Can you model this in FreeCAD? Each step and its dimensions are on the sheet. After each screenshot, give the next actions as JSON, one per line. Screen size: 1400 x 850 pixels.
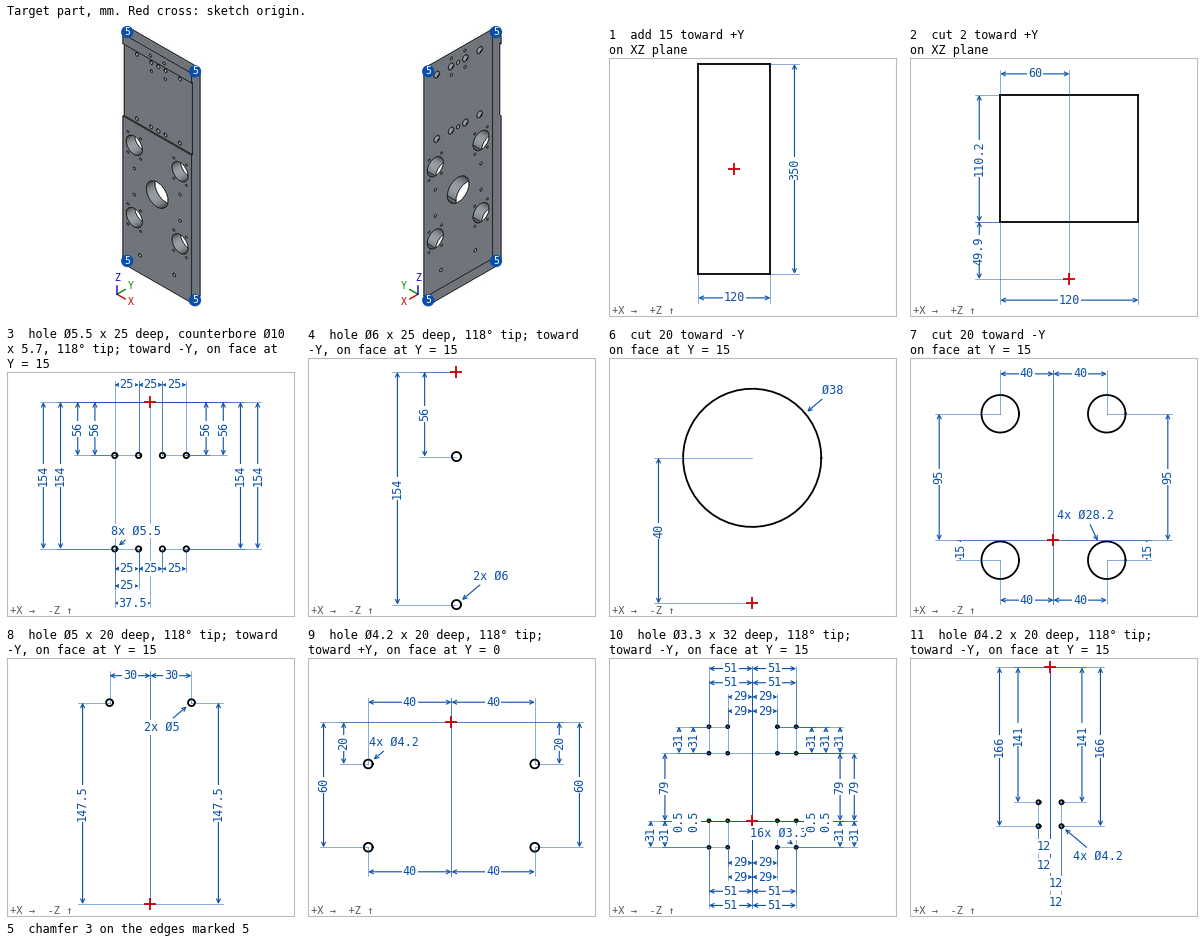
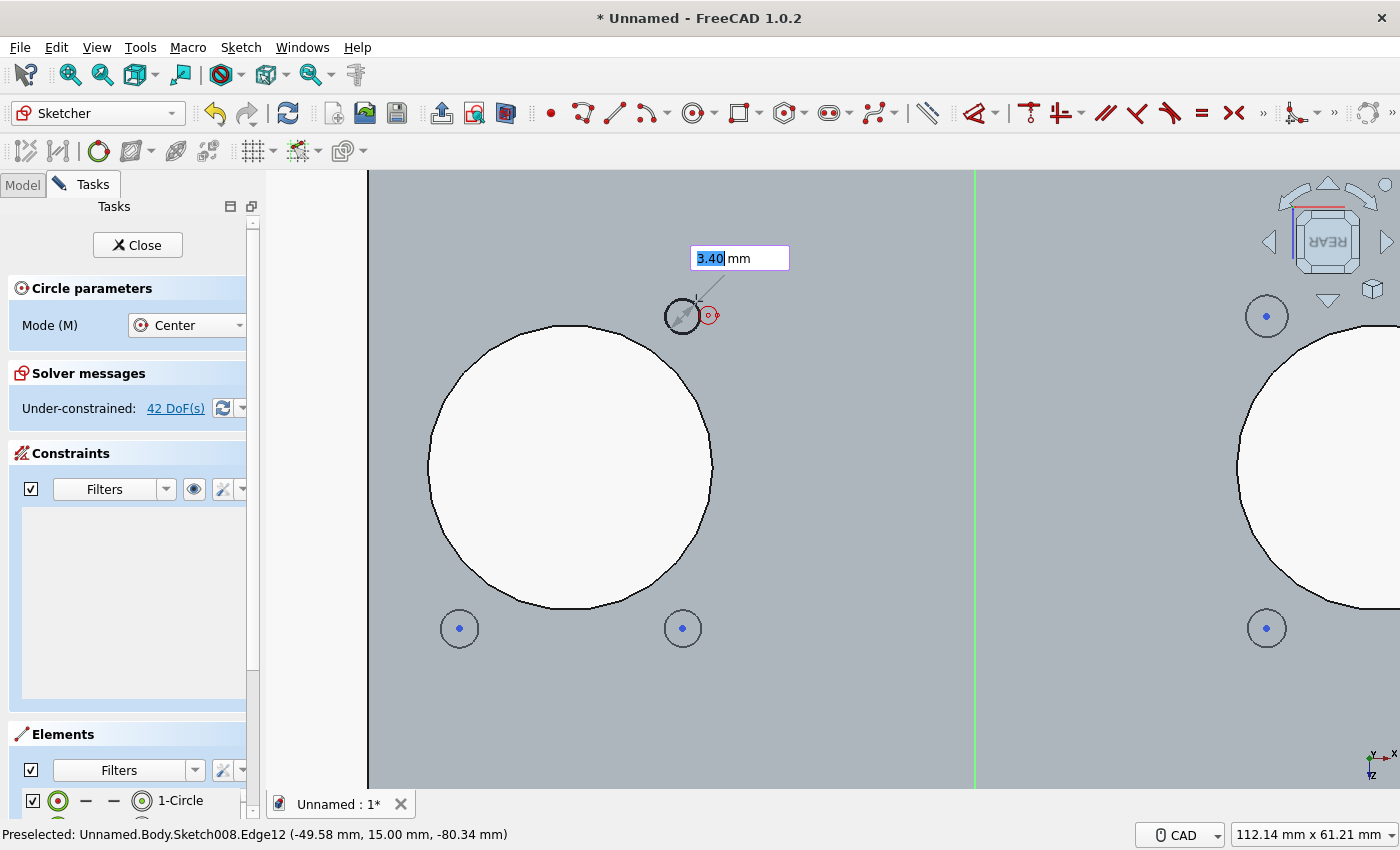
{"action": "left_click", "coordinate": [693, 299]}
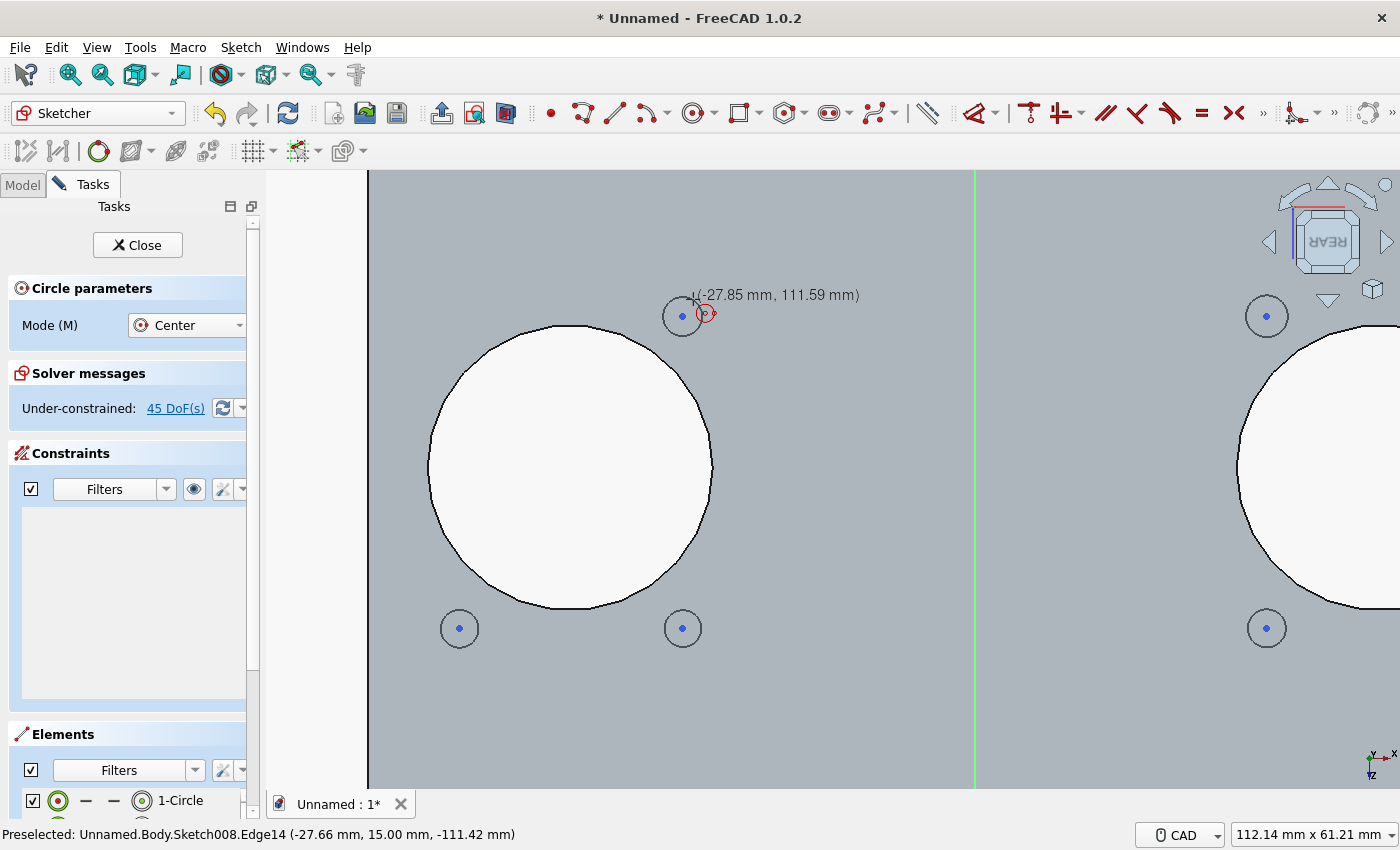
{"action": "scroll", "coordinate": [459, 311], "scroll_direction": "up", "scroll_amount": 2}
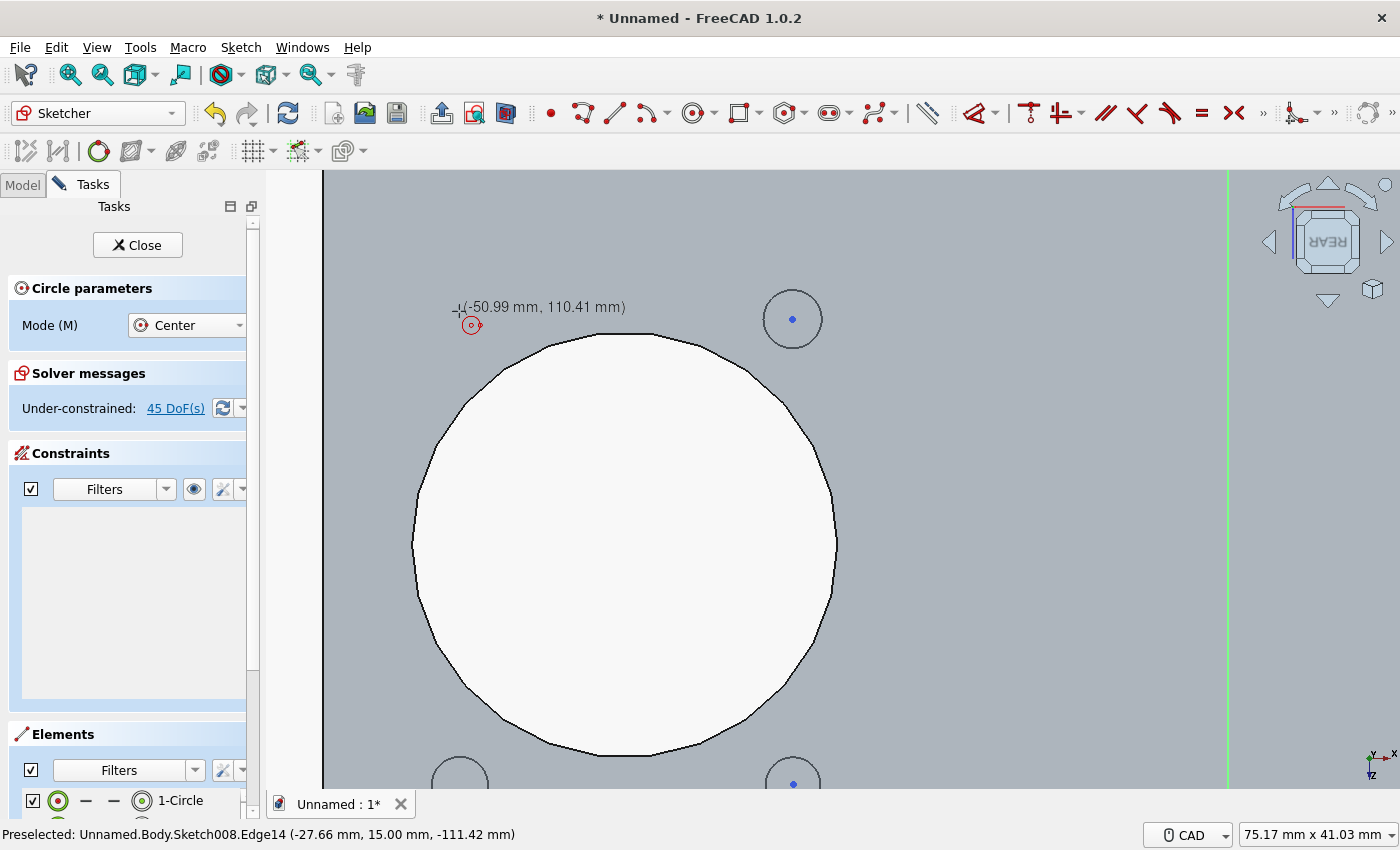
{"action": "scroll", "coordinate": [673, 302], "scroll_direction": "down", "scroll_amount": 9}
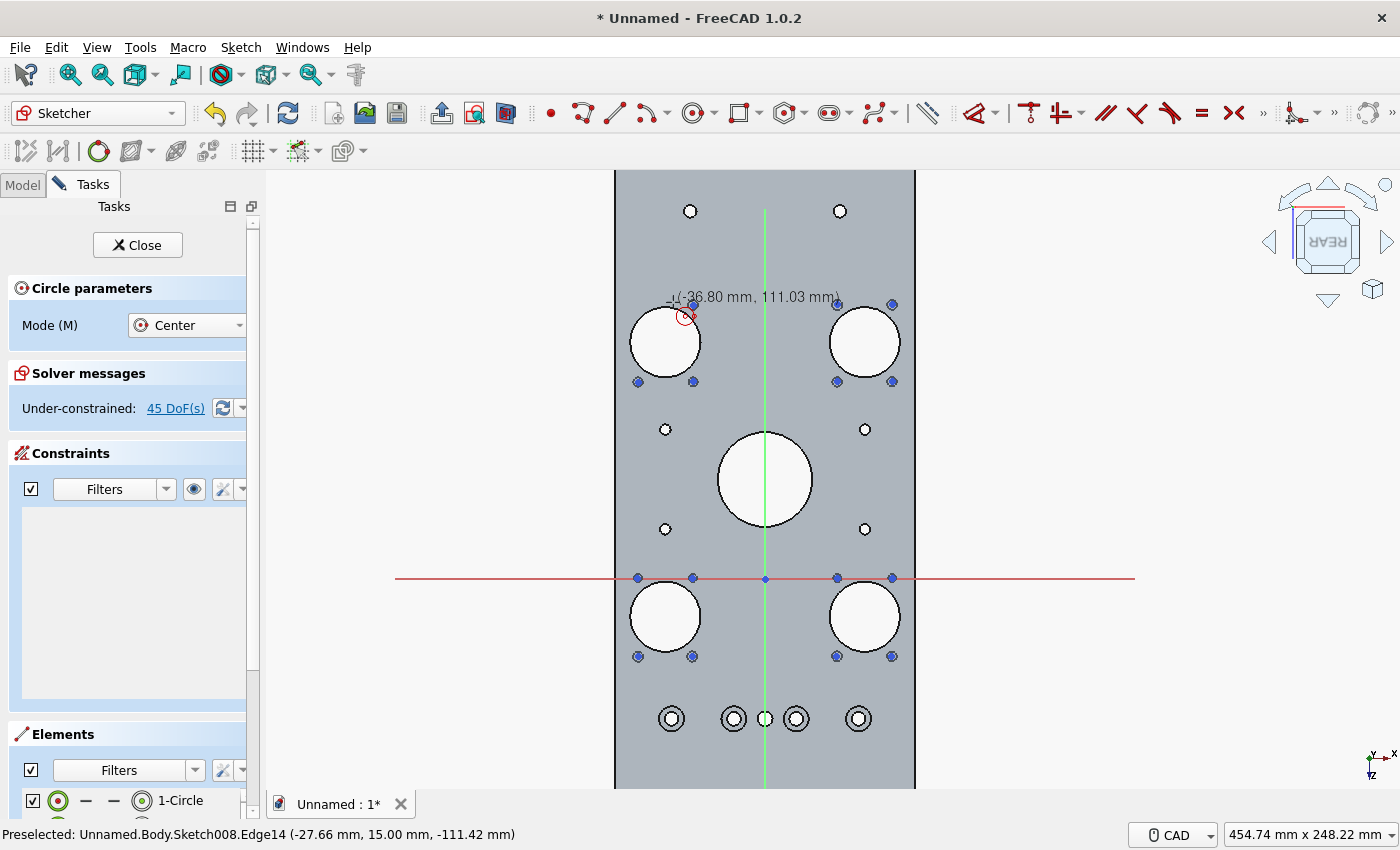
{"action": "left_click", "coordinate": [638, 304]}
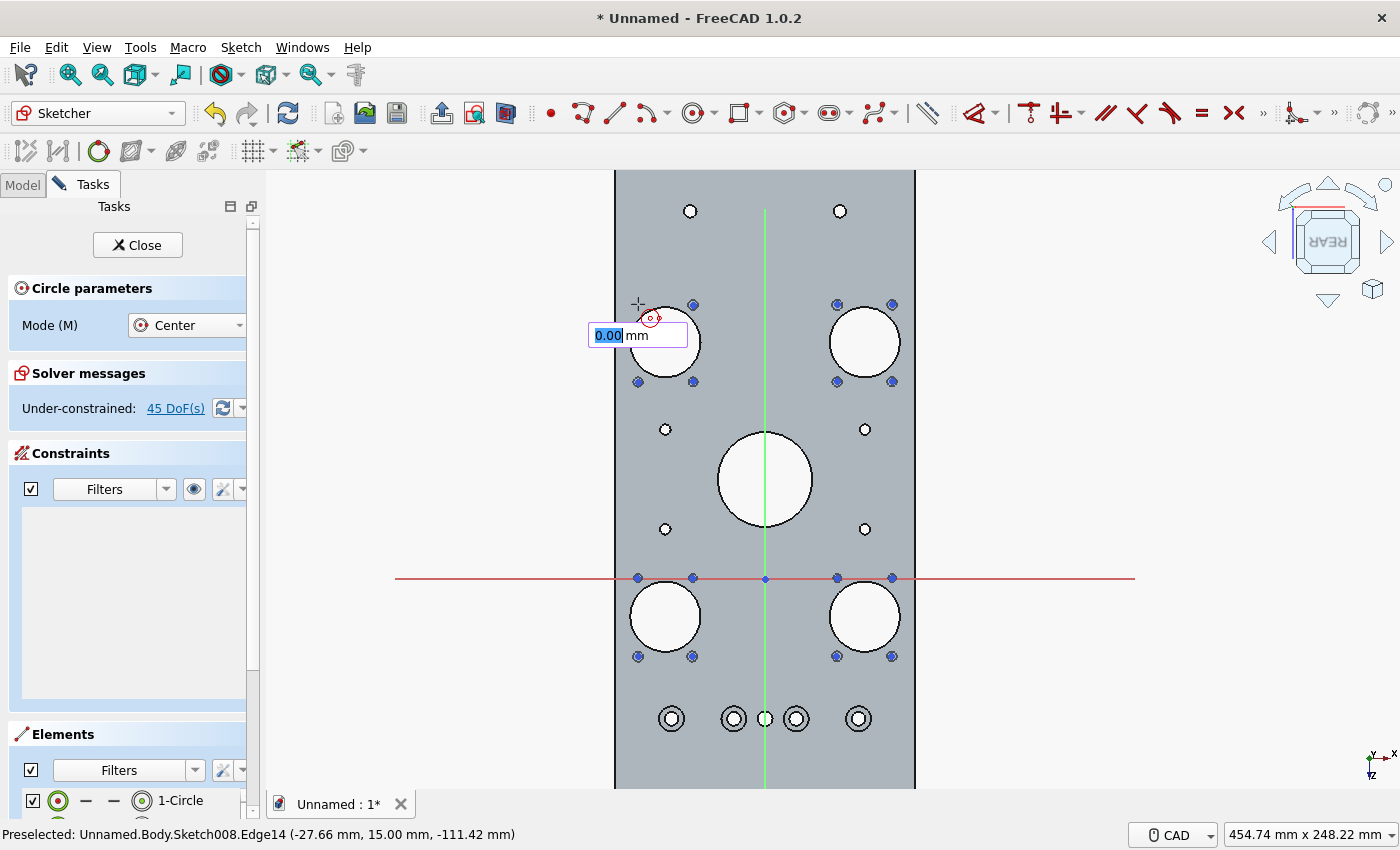
{"action": "scroll", "coordinate": [641, 301], "scroll_direction": "up", "scroll_amount": 7}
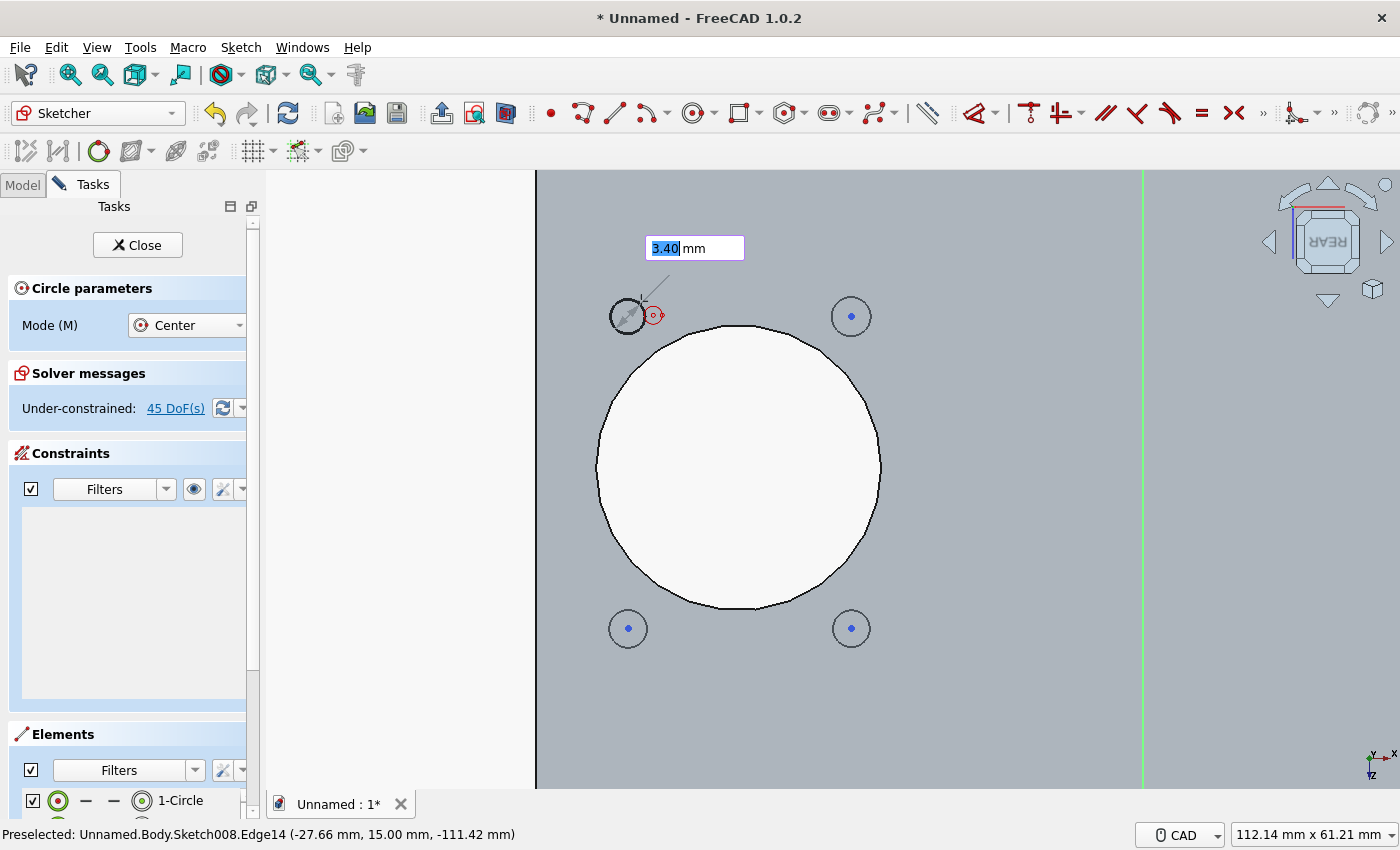
{"action": "left_click", "coordinate": [639, 299]}
{"action": "key", "text": "Escape"}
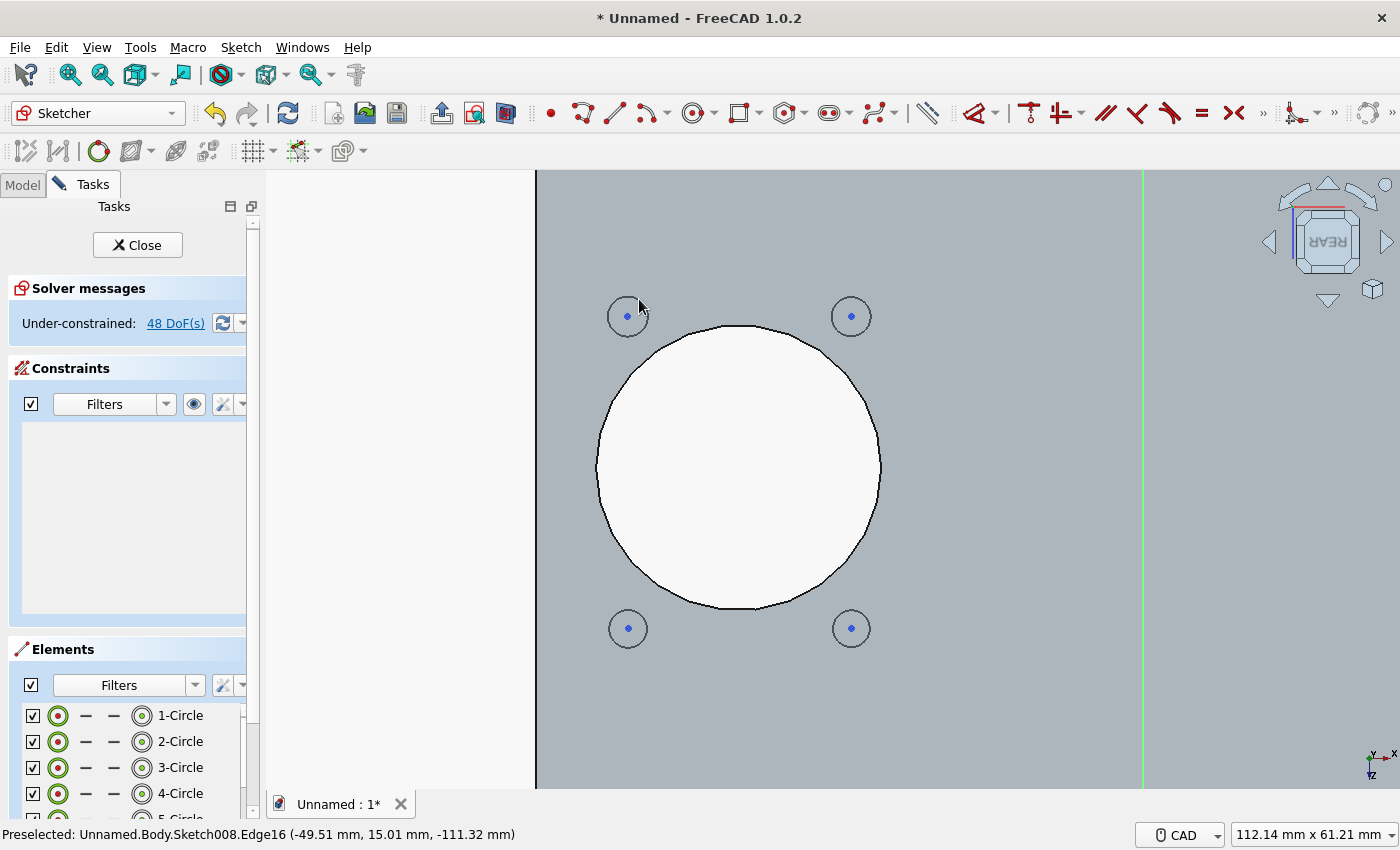
{"action": "scroll", "coordinate": [641, 301], "scroll_direction": "down", "scroll_amount": 7}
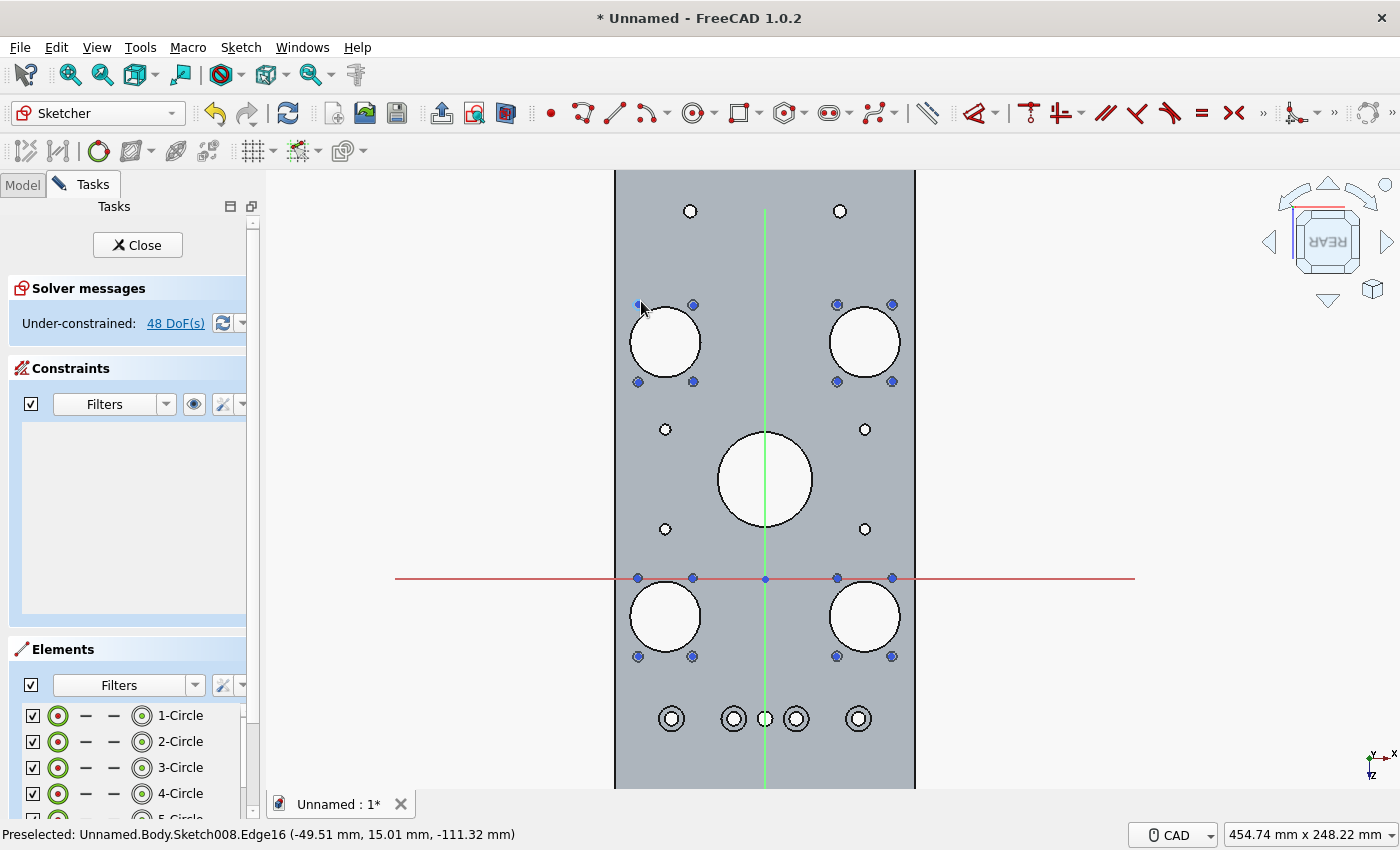
{"action": "scroll", "coordinate": [895, 653], "scroll_direction": "up", "scroll_amount": 6}